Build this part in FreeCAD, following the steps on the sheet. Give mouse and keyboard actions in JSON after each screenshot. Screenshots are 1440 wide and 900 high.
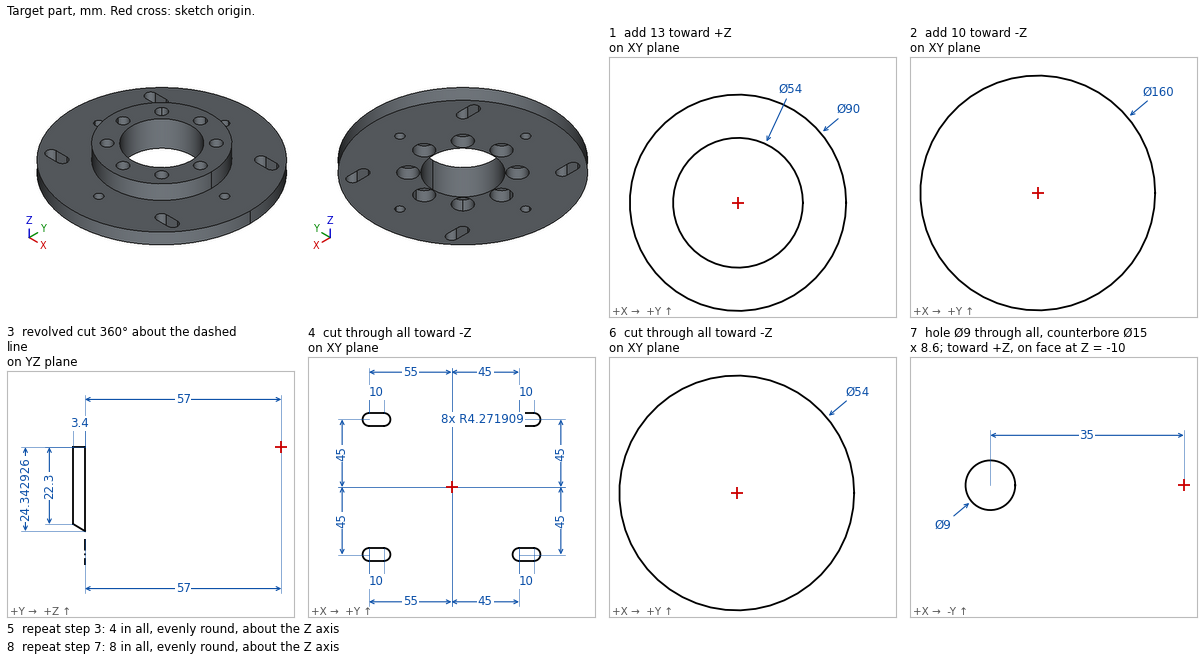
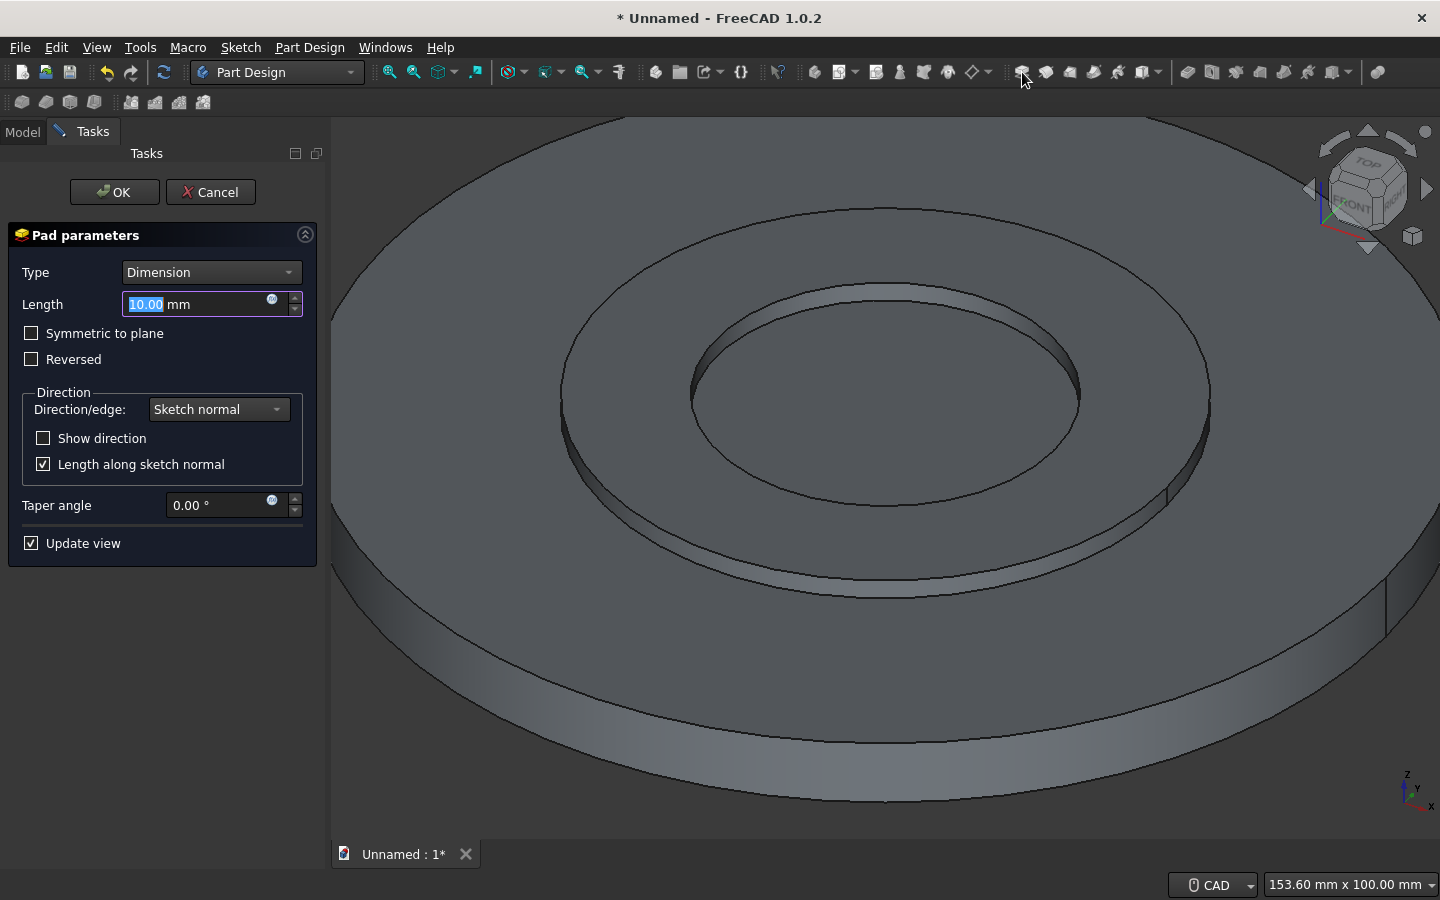
{"action": "type", "text": "10"}
{"action": "key", "text": "Tab"}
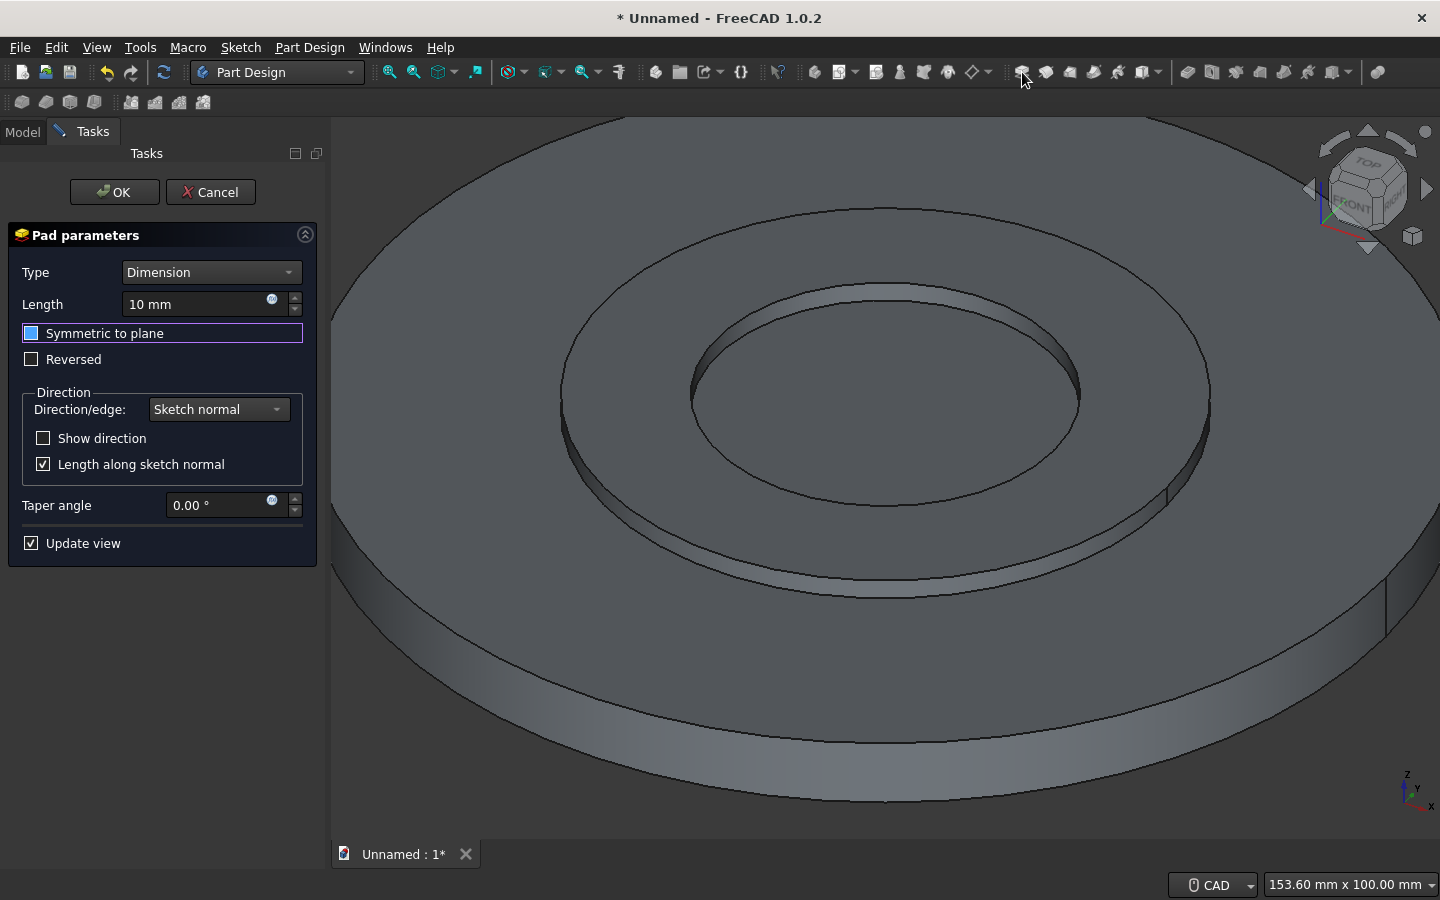
{"action": "left_click", "coordinate": [30, 359]}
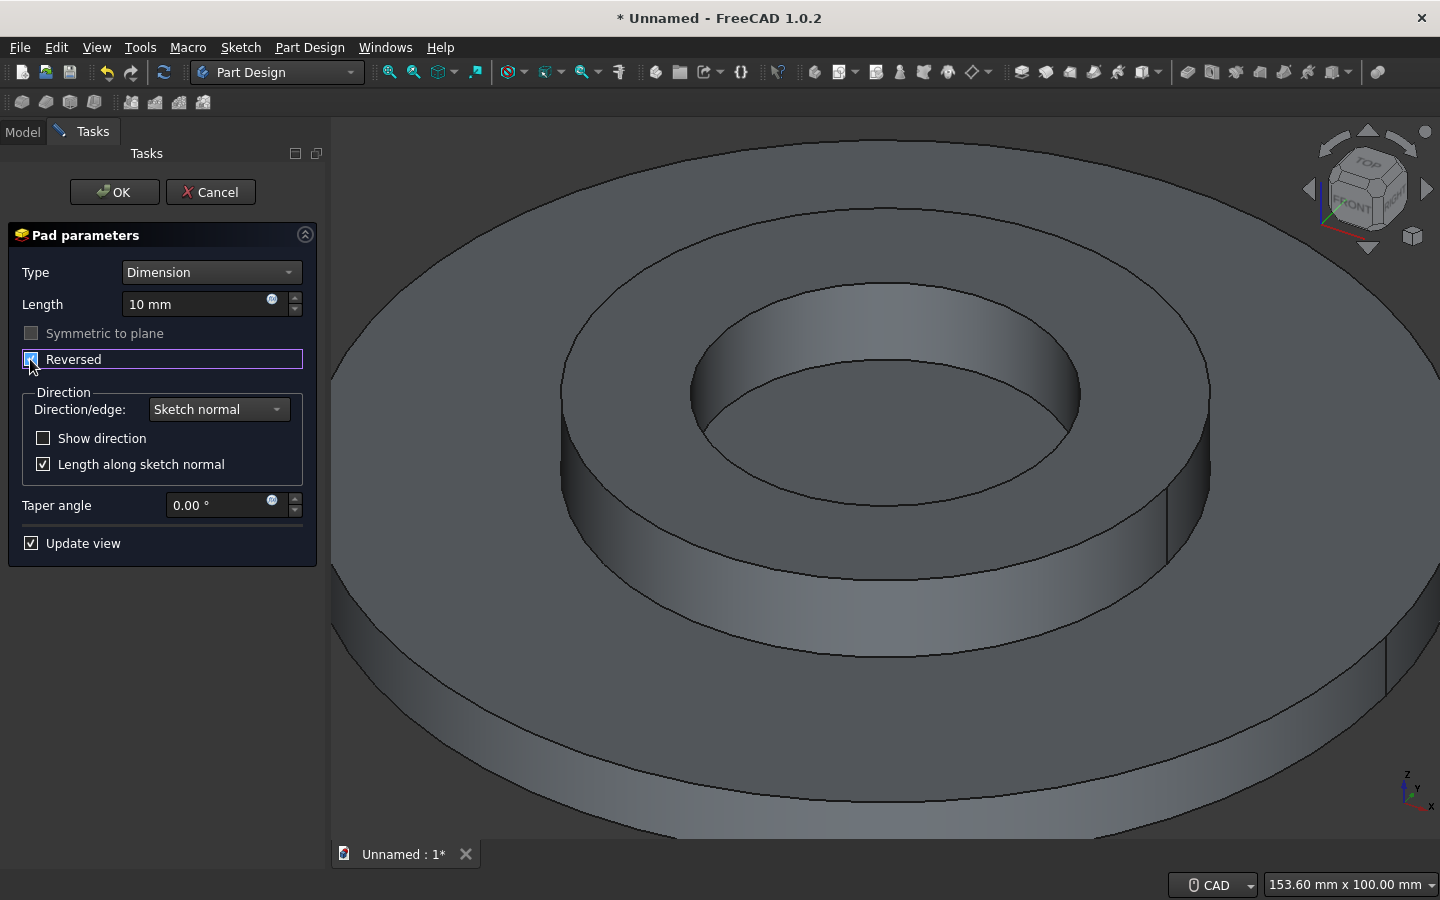
{"action": "left_click", "coordinate": [115, 192]}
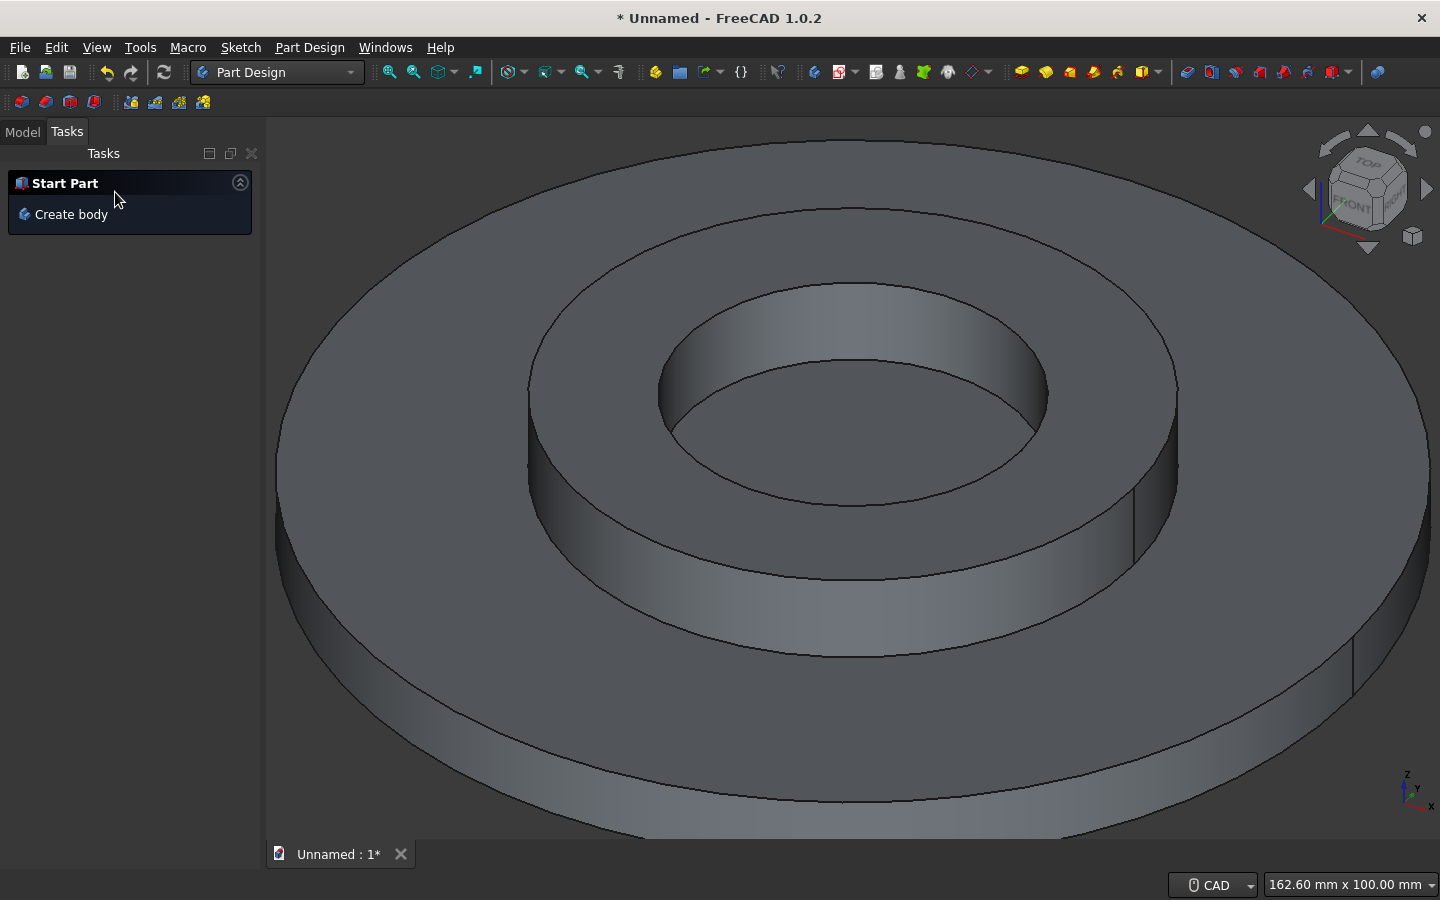
{"action": "left_click", "coordinate": [390, 72]}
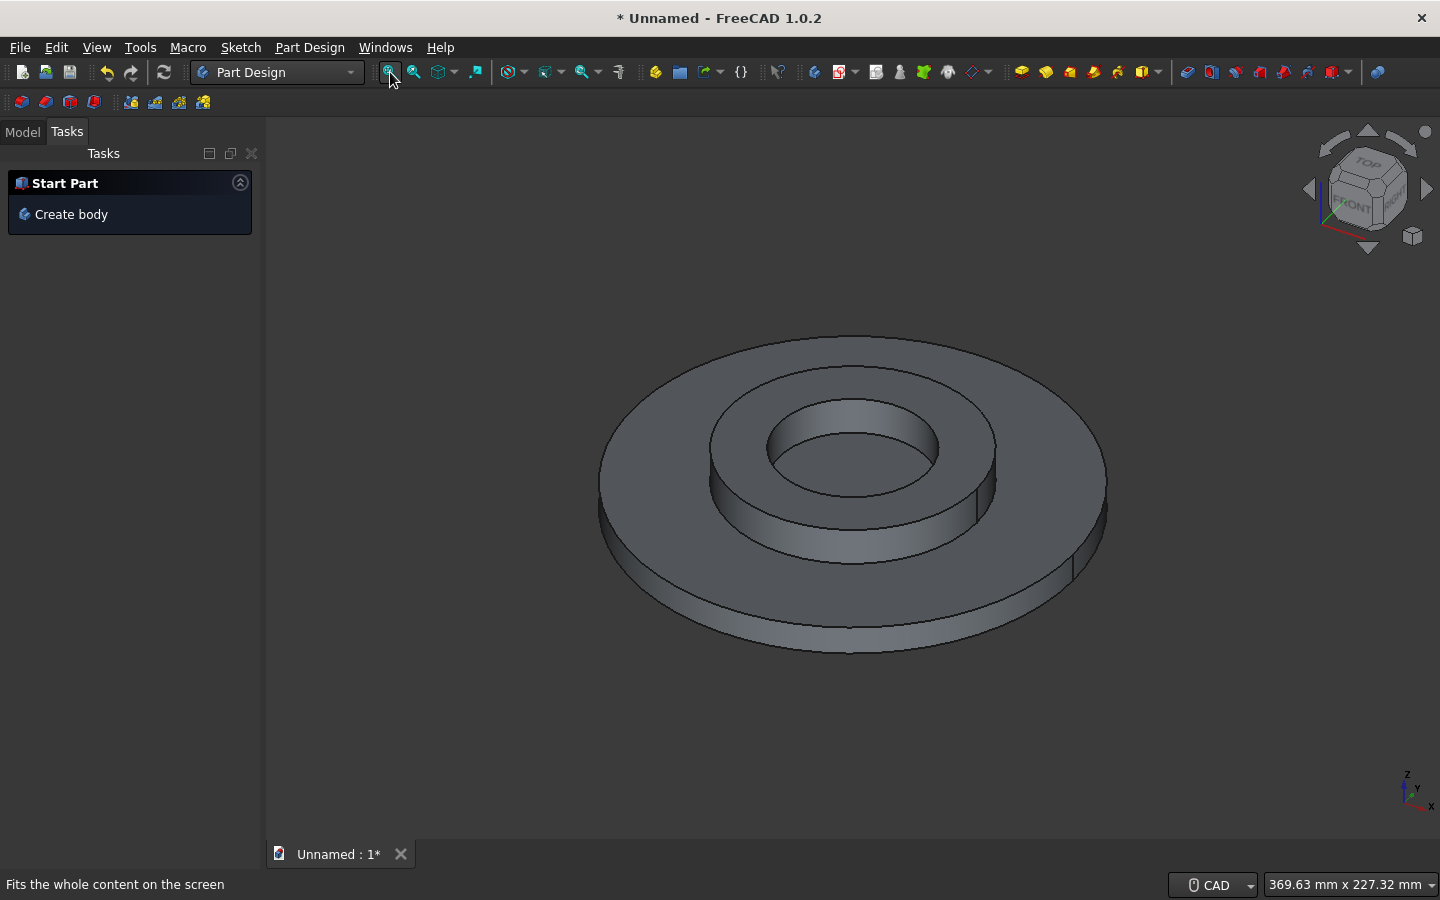
{"action": "left_click", "coordinate": [840, 72]}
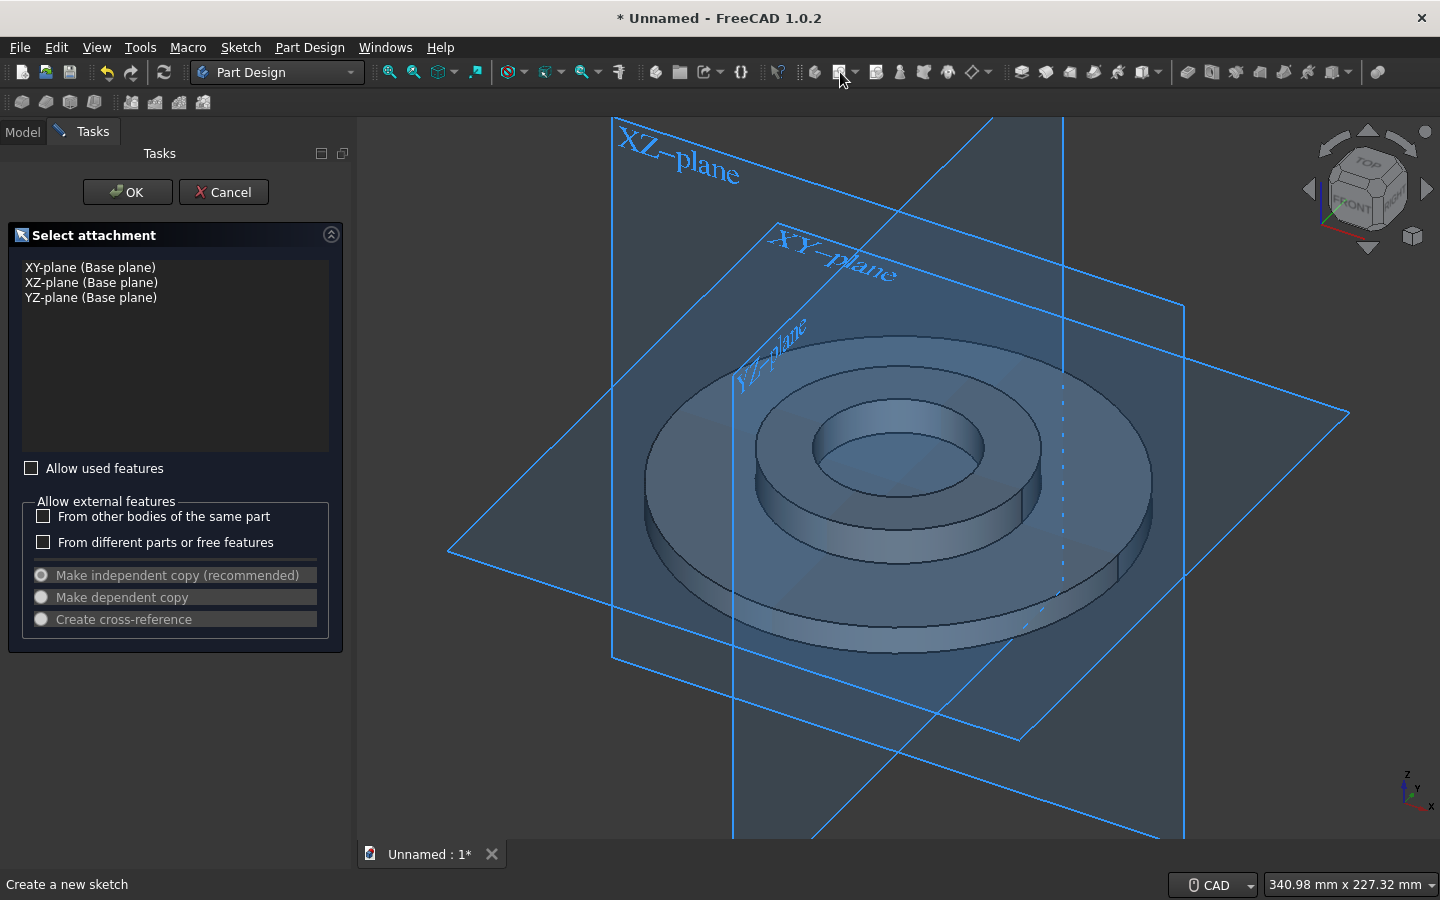
{"action": "left_click", "coordinate": [82, 298]}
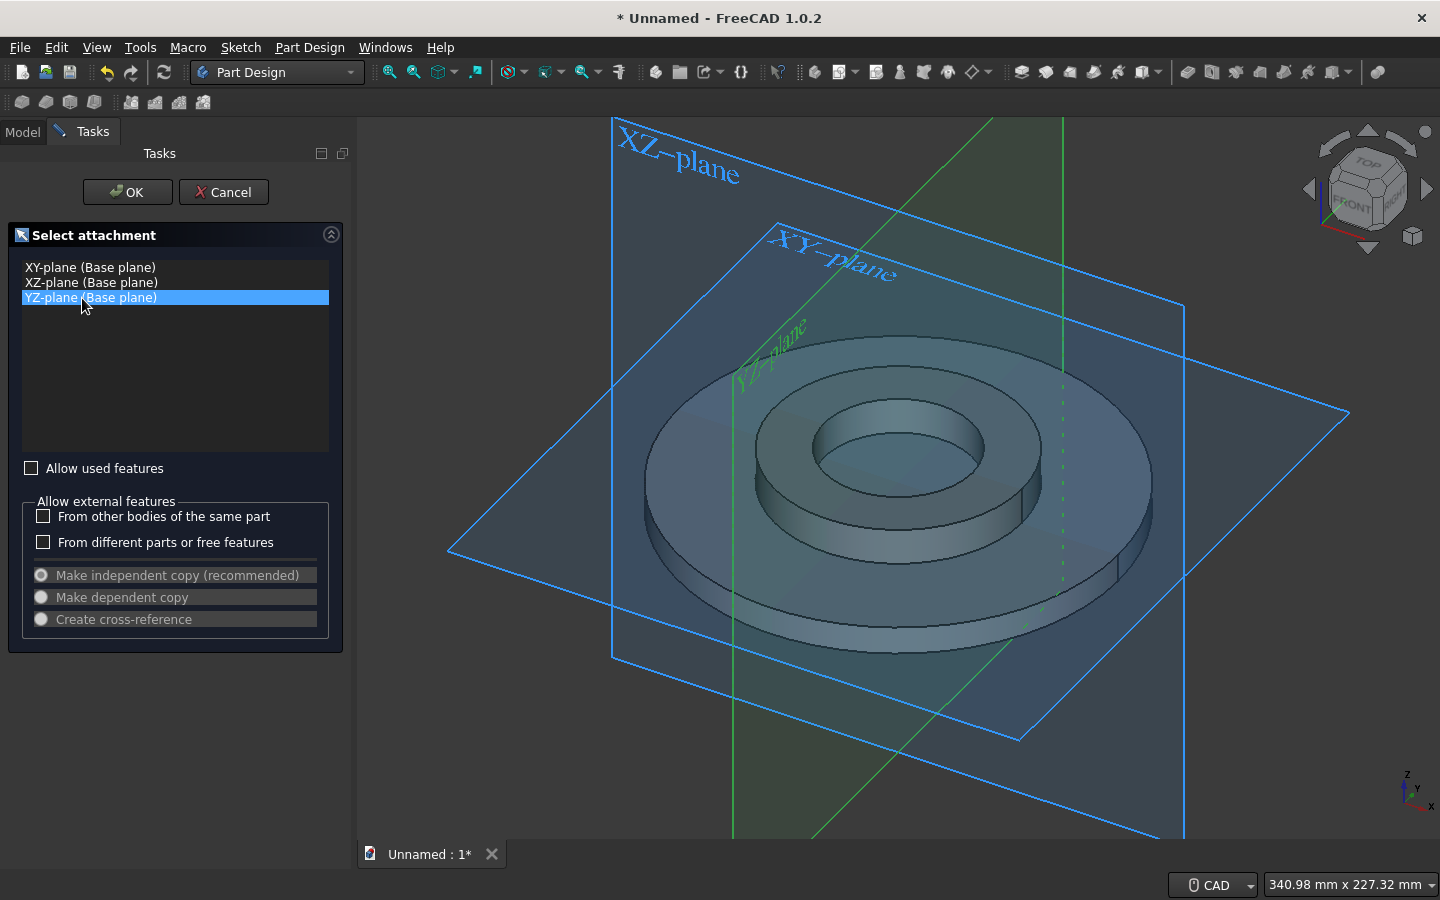
{"action": "left_click", "coordinate": [128, 192]}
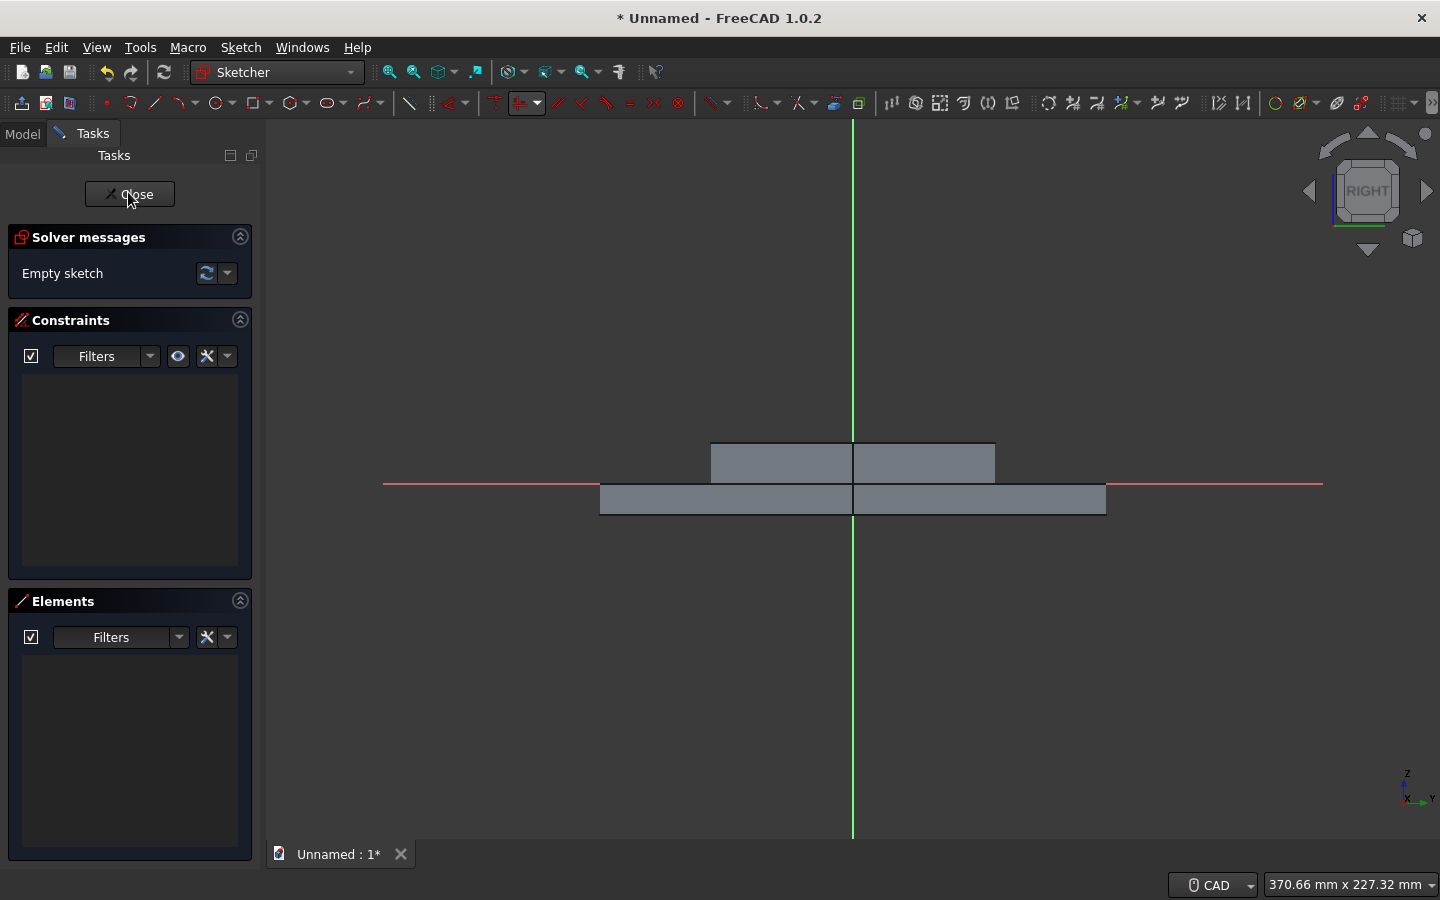
{"action": "key", "text": "q s"}